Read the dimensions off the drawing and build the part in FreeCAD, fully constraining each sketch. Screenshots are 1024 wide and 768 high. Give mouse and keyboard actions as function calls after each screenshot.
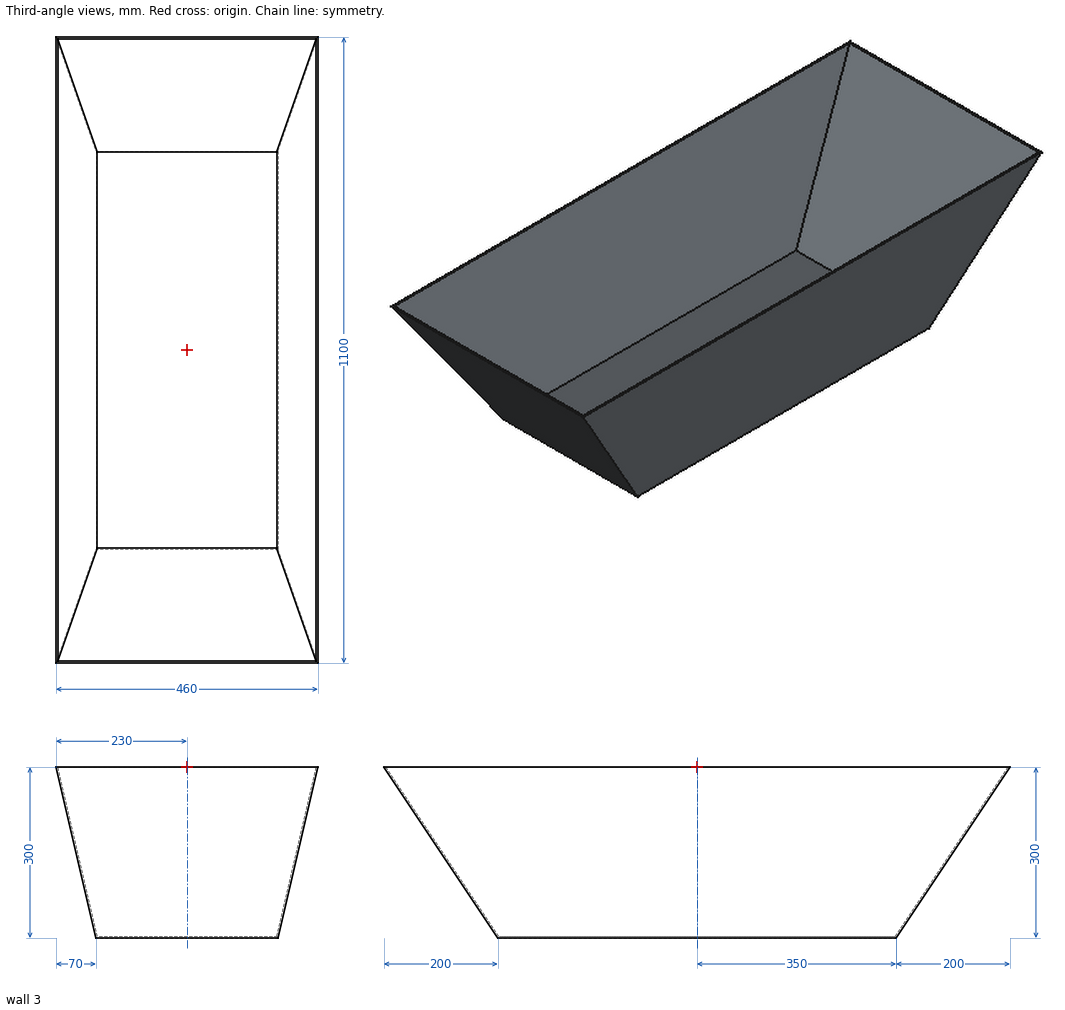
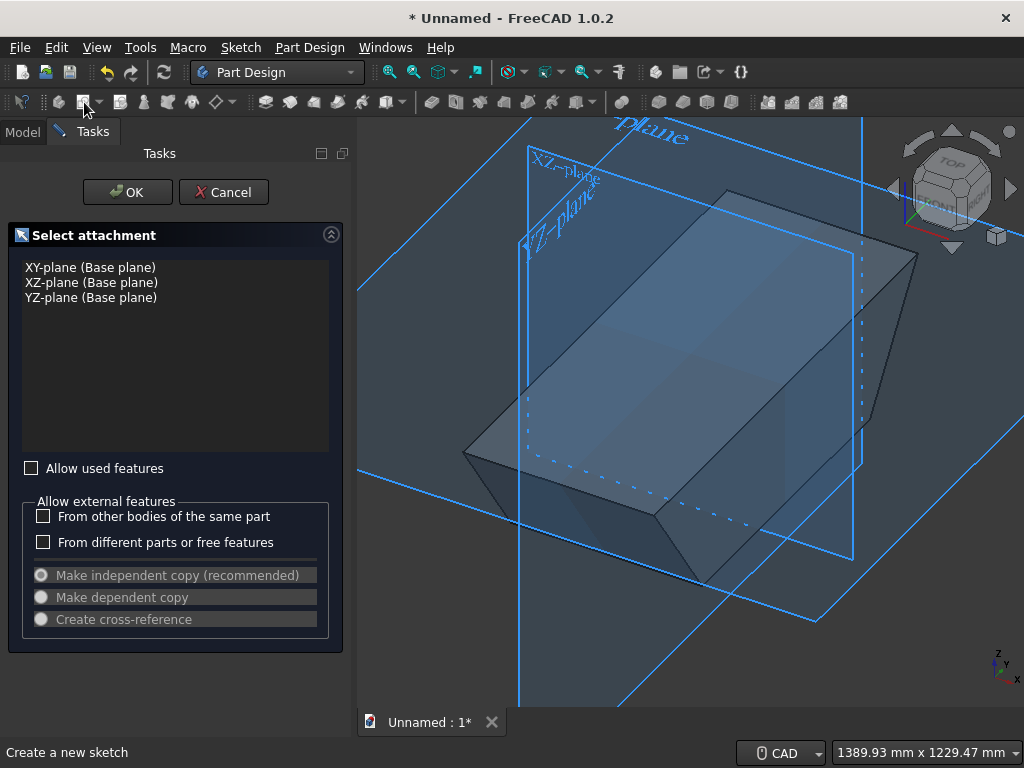
click(82, 282)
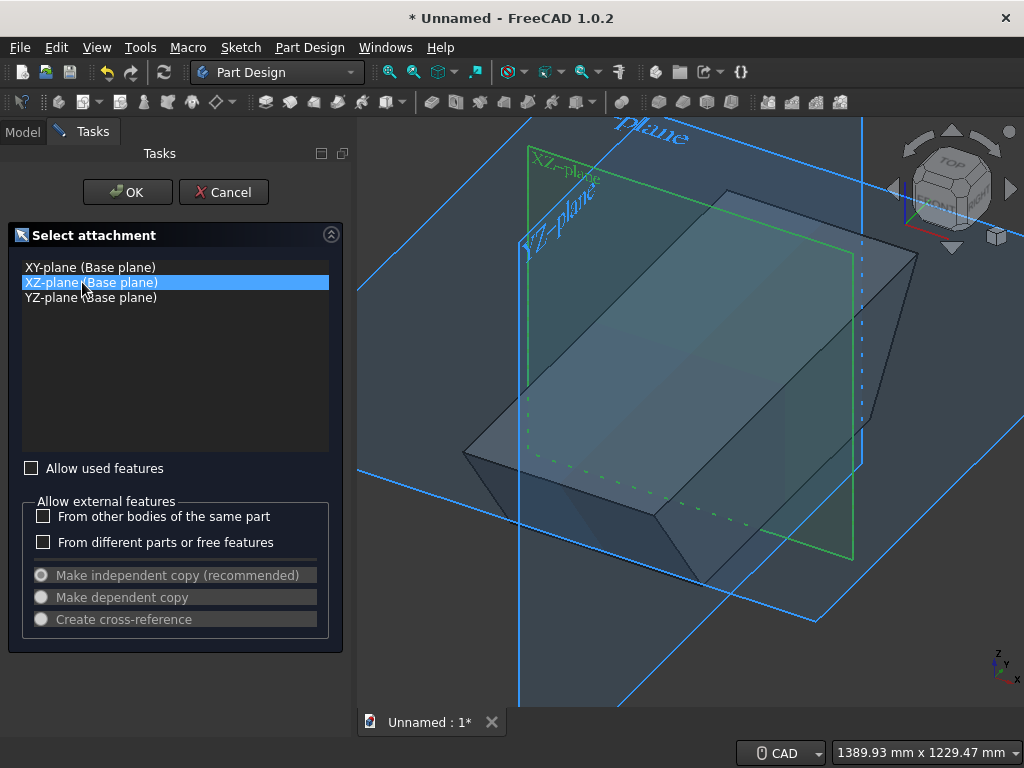
click(128, 192)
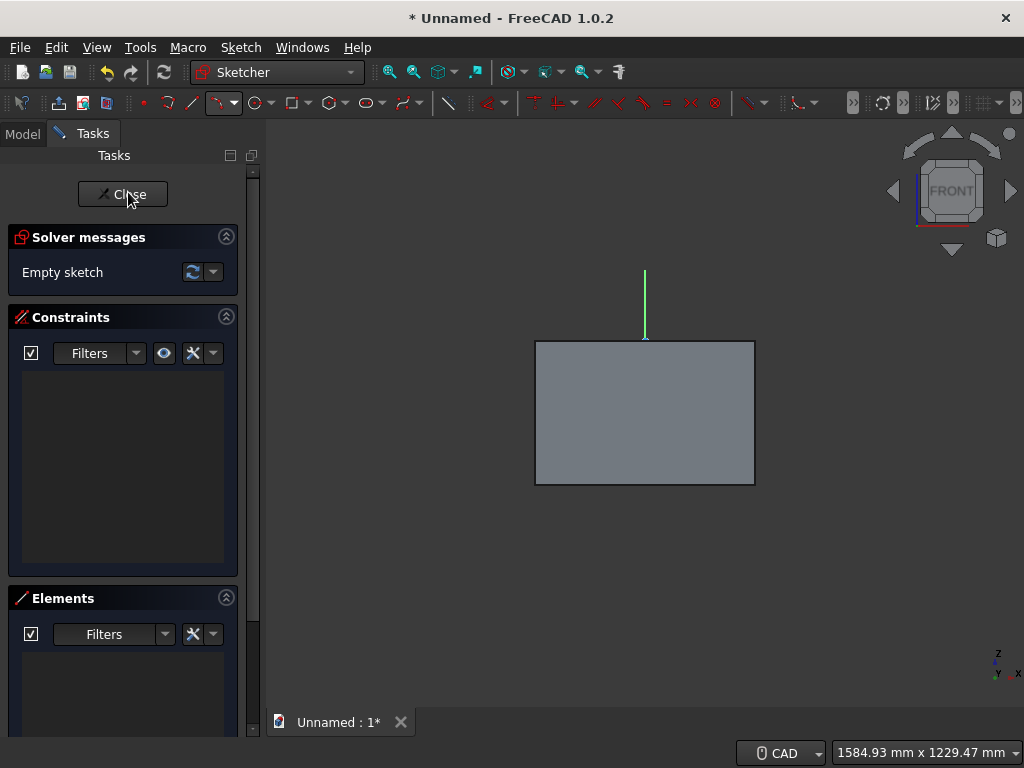
key(q)
key(s)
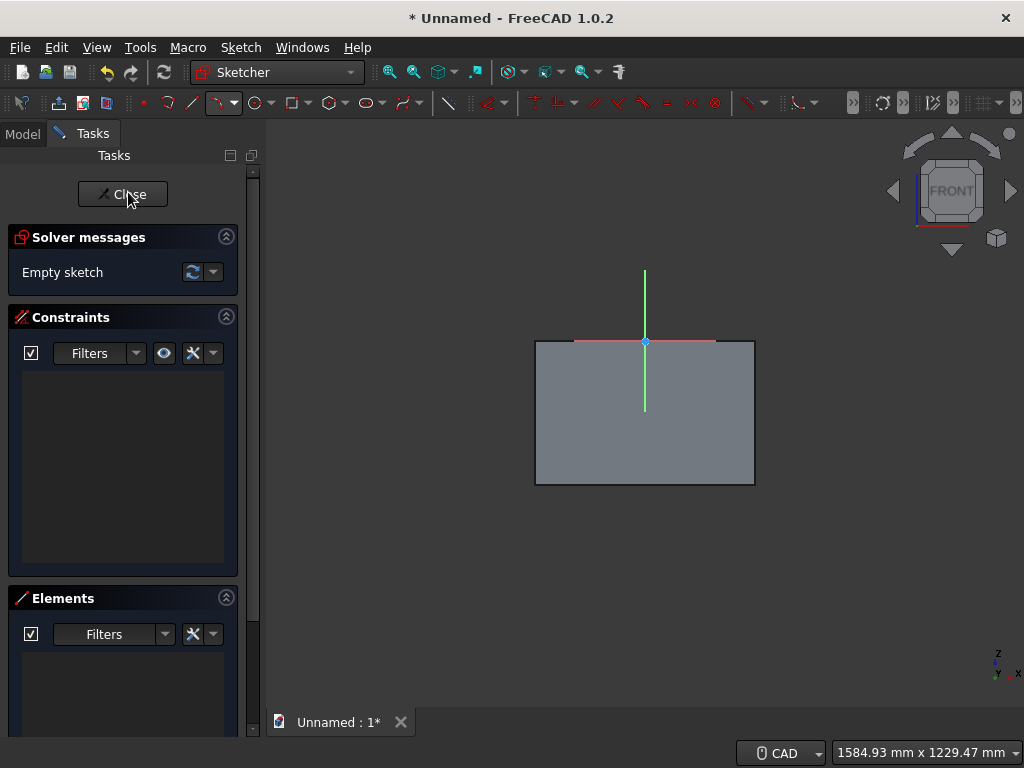
scroll(728, 413, up, 3)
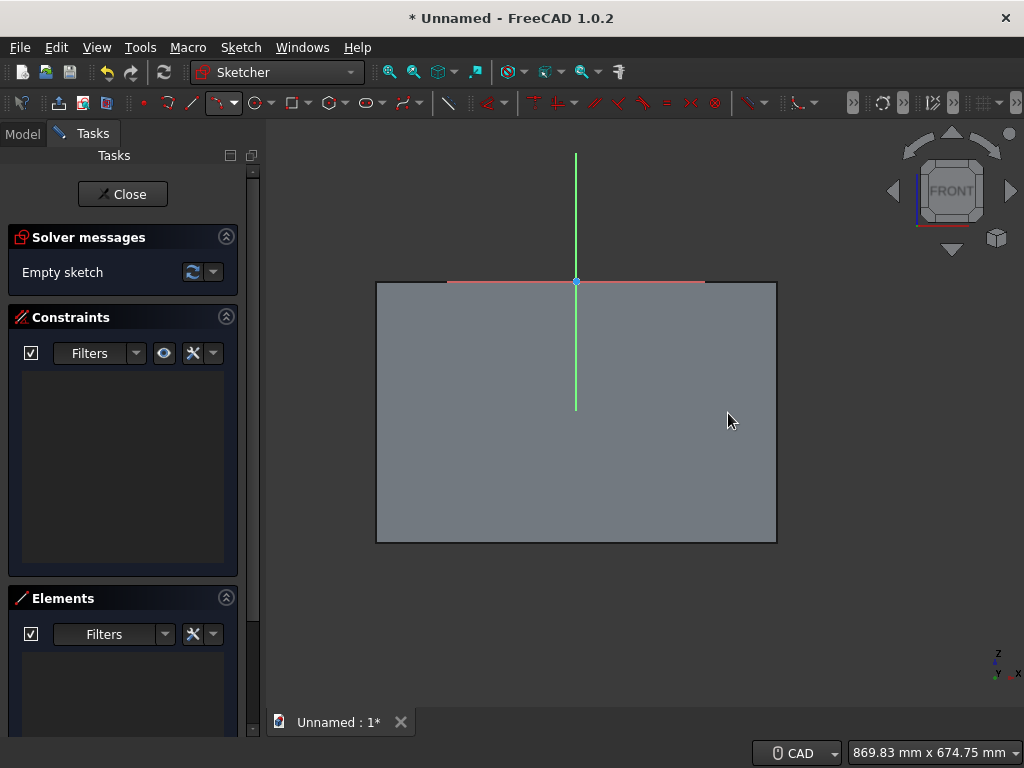
click(168, 104)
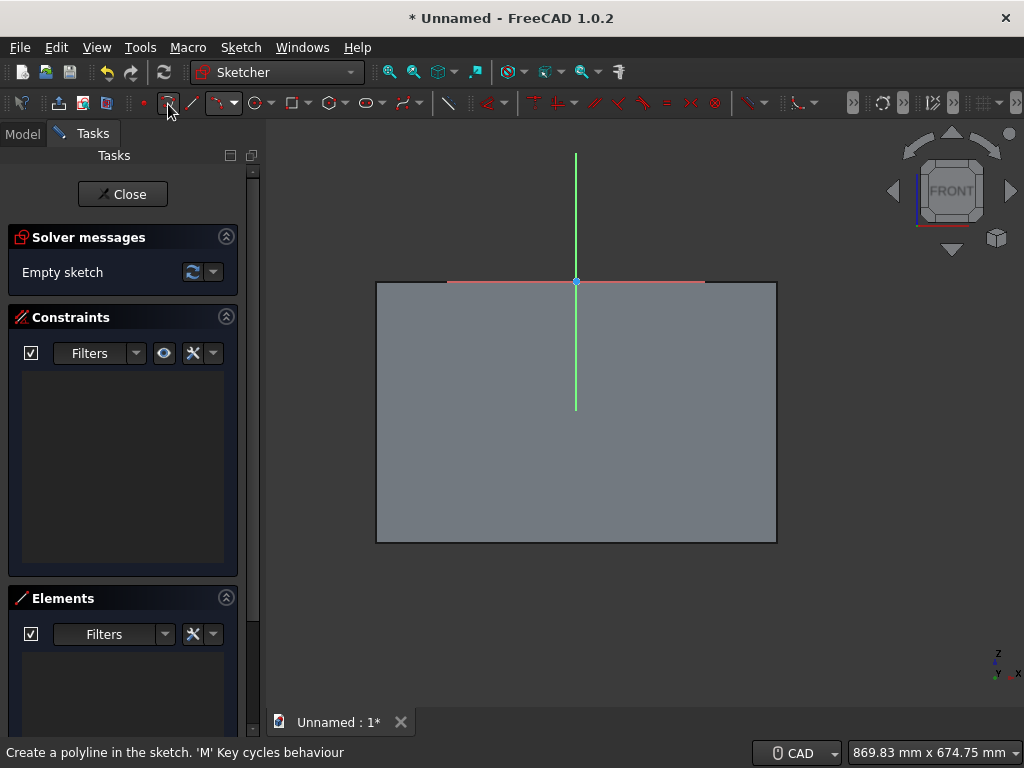
click(376, 282)
click(437, 543)
click(376, 543)
click(376, 283)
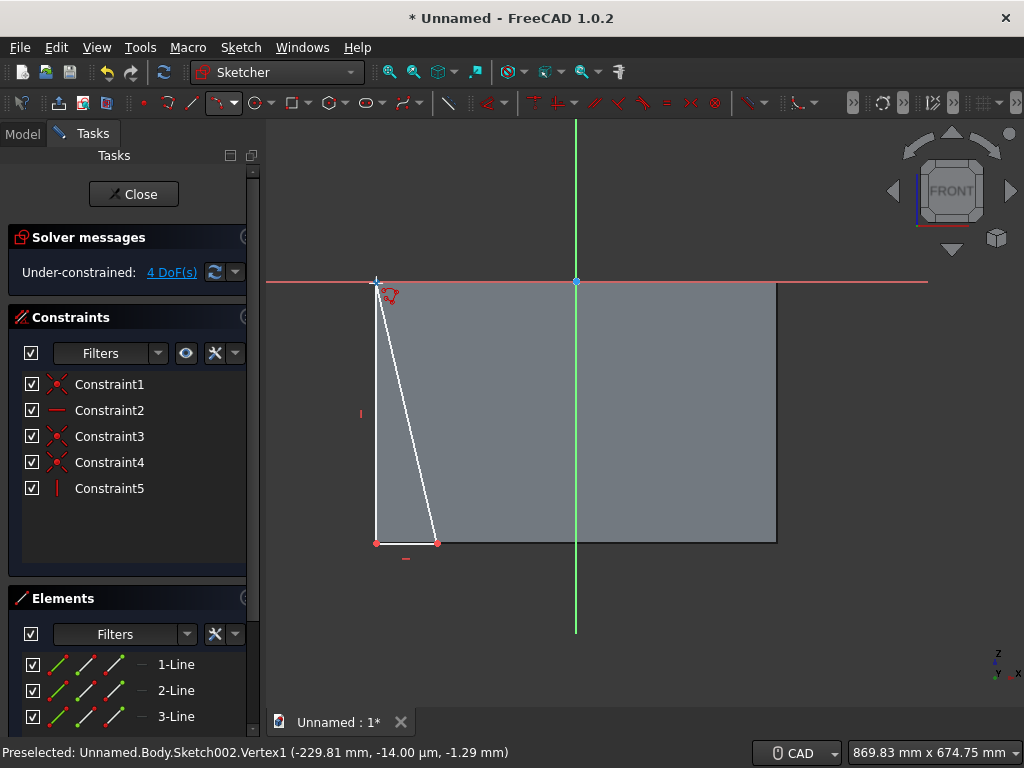
click(777, 282)
click(777, 543)
click(716, 543)
click(777, 282)
key(Escape)
key(Escape)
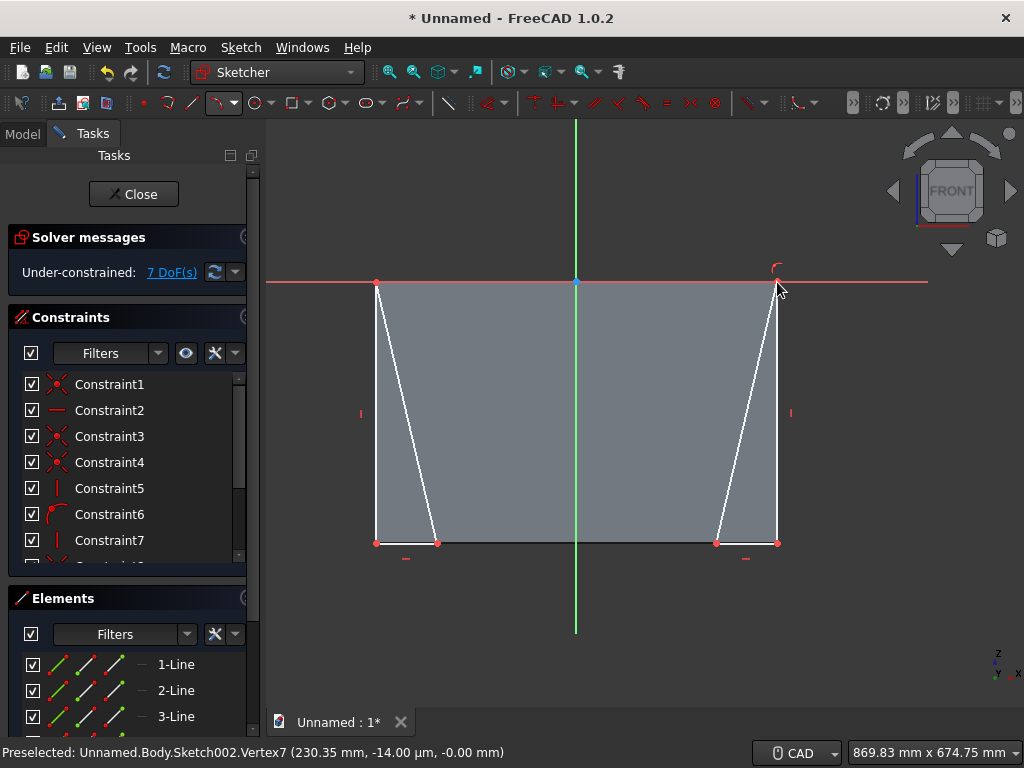
click(376, 283)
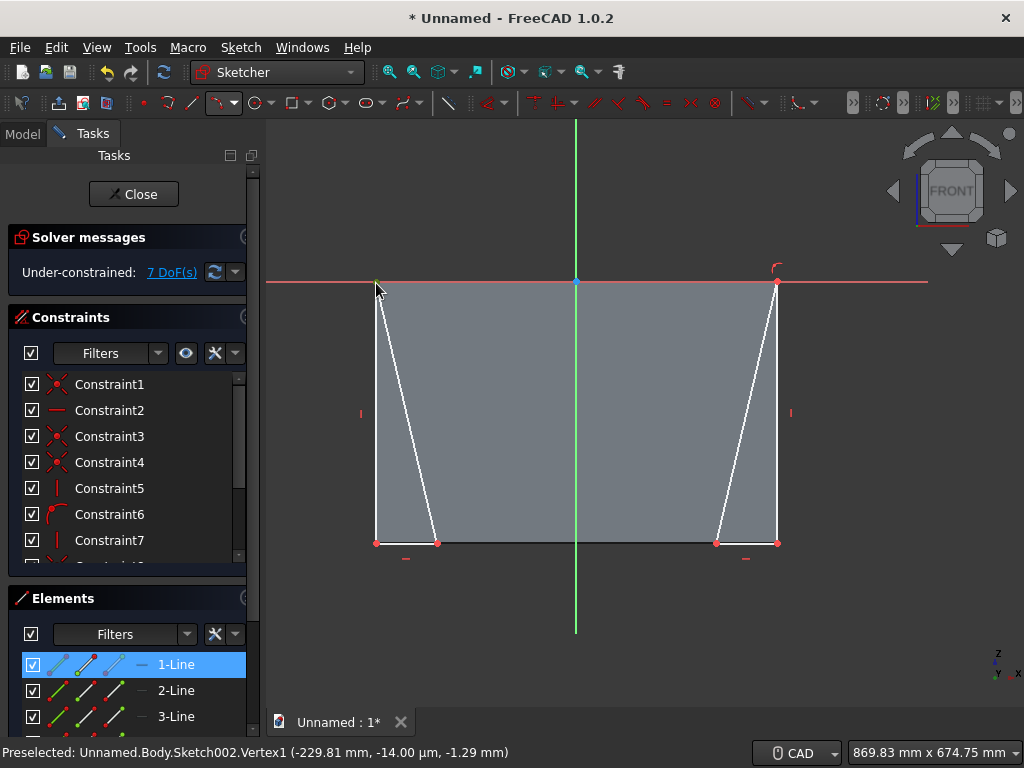
click(777, 282)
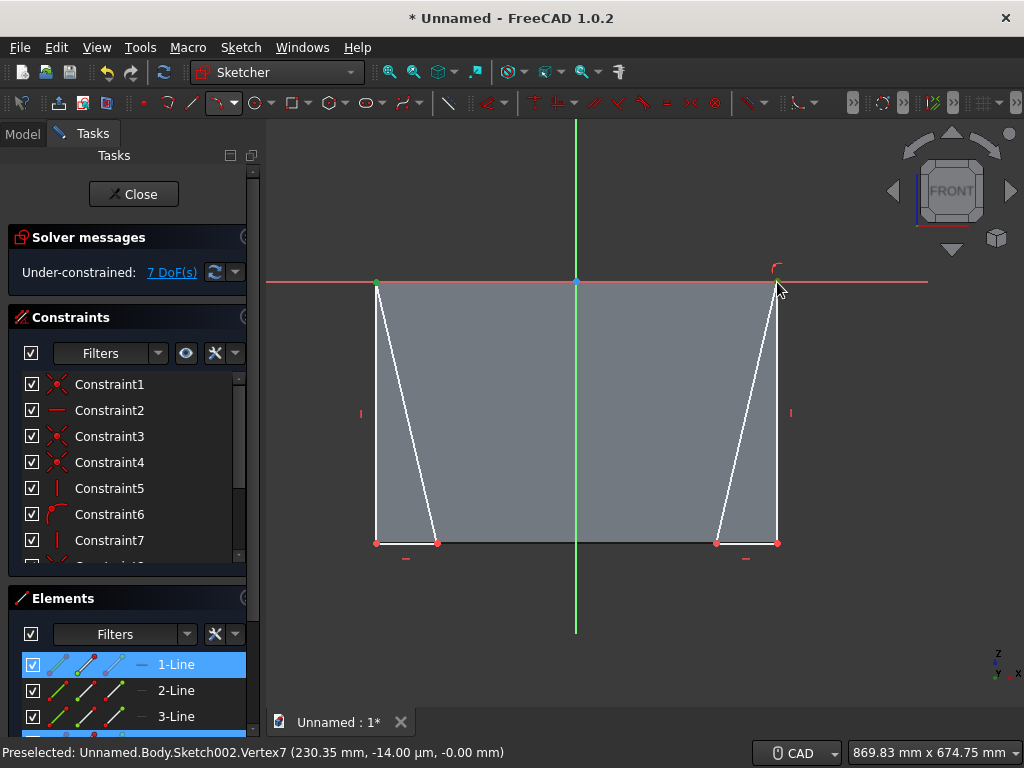
click(576, 603)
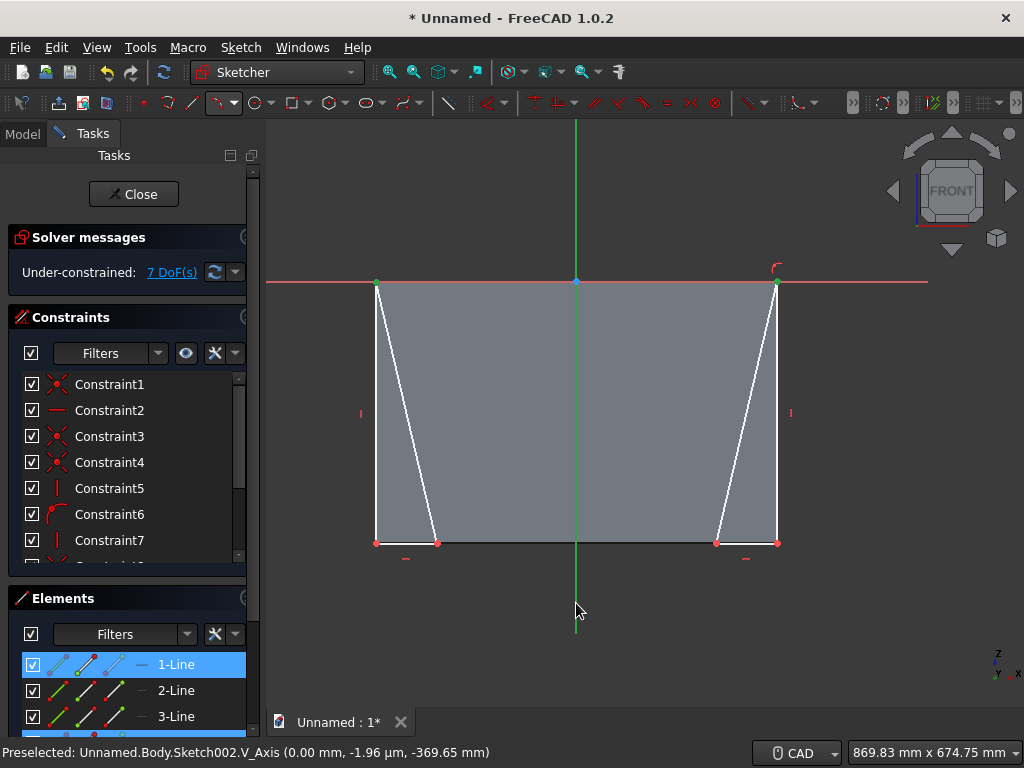
click(692, 104)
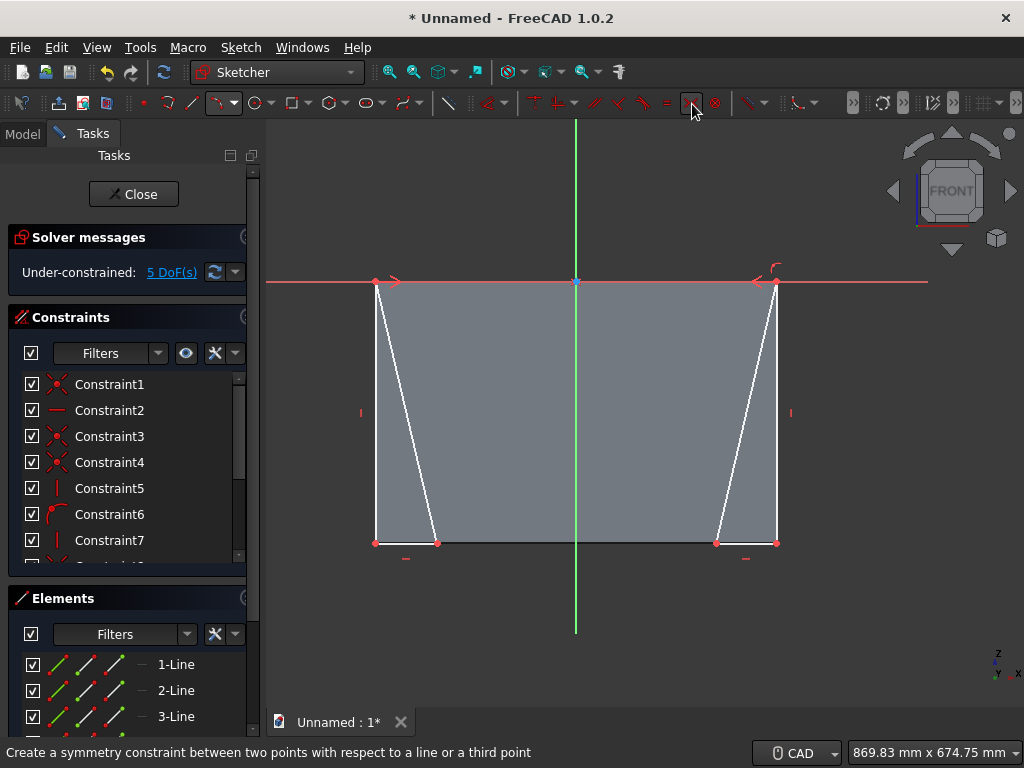
click(437, 544)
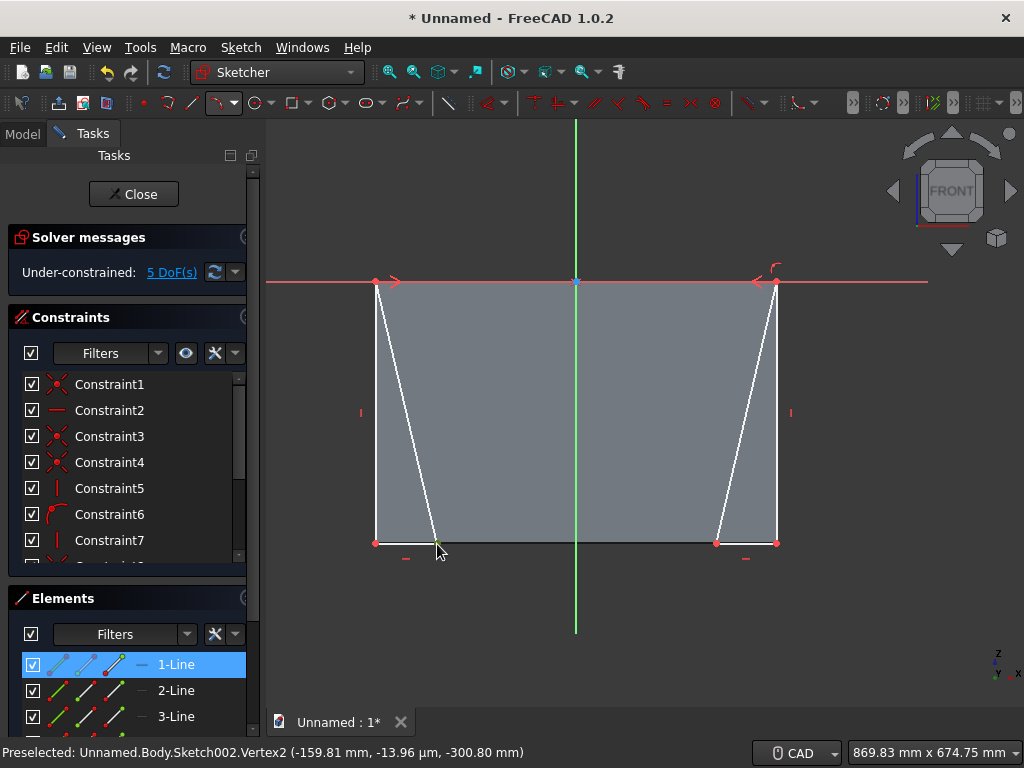
click(716, 544)